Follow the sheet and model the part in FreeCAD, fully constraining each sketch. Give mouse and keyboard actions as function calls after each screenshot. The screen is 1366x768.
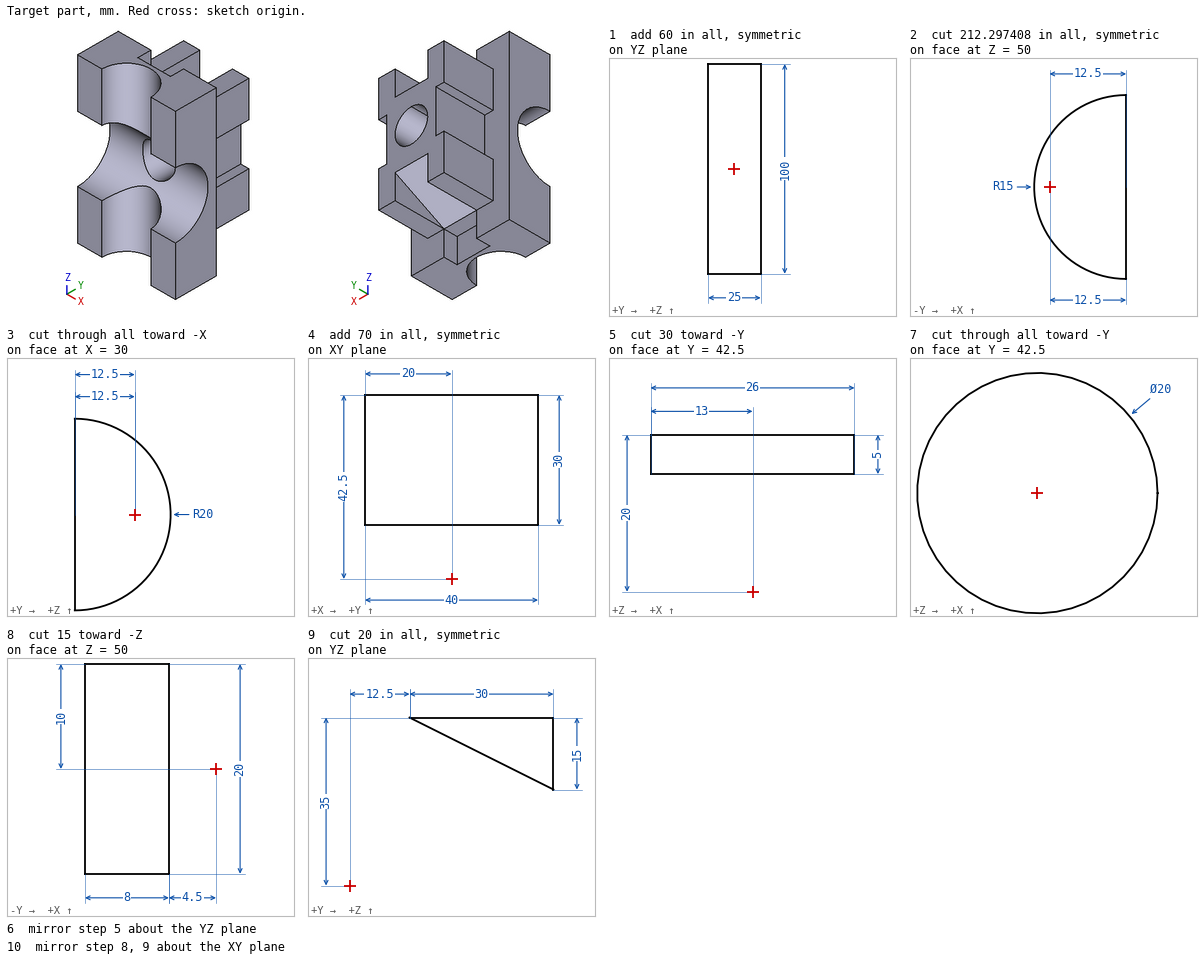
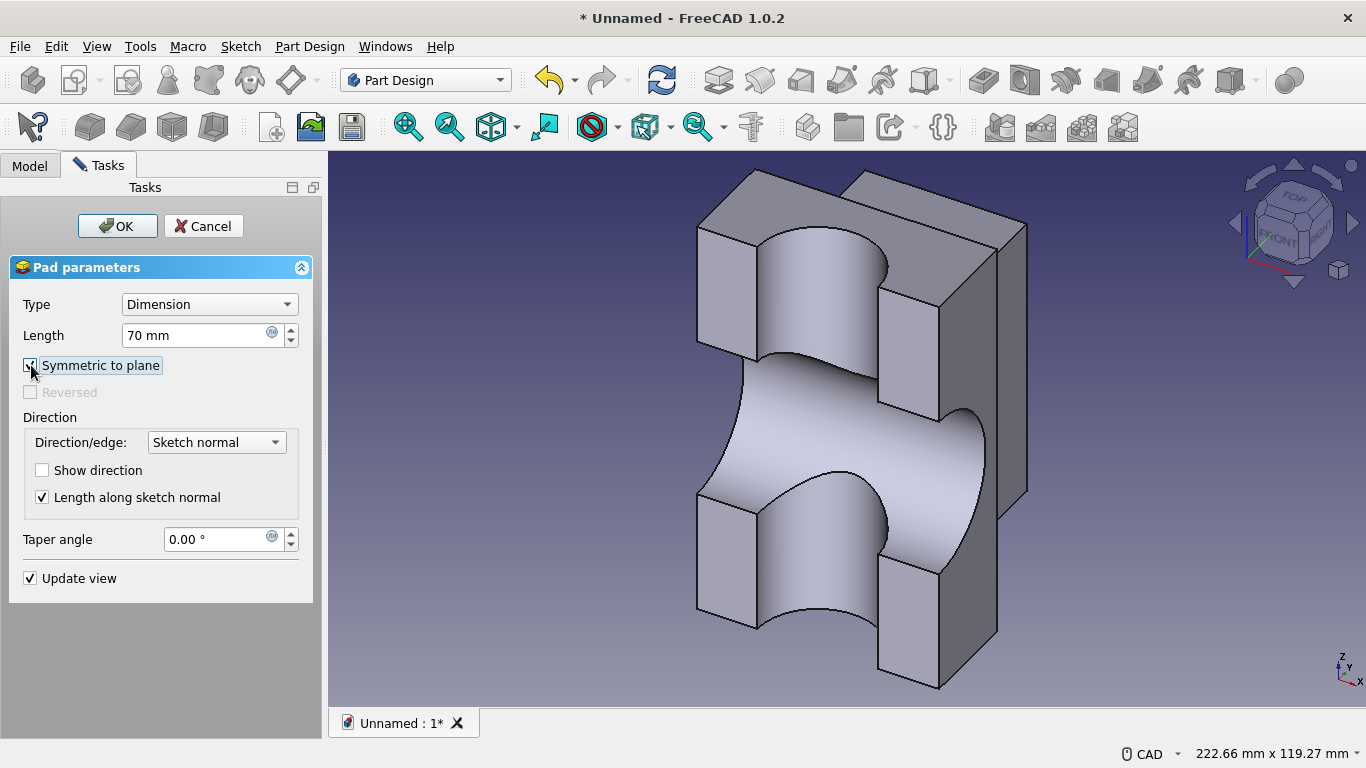
click(118, 226)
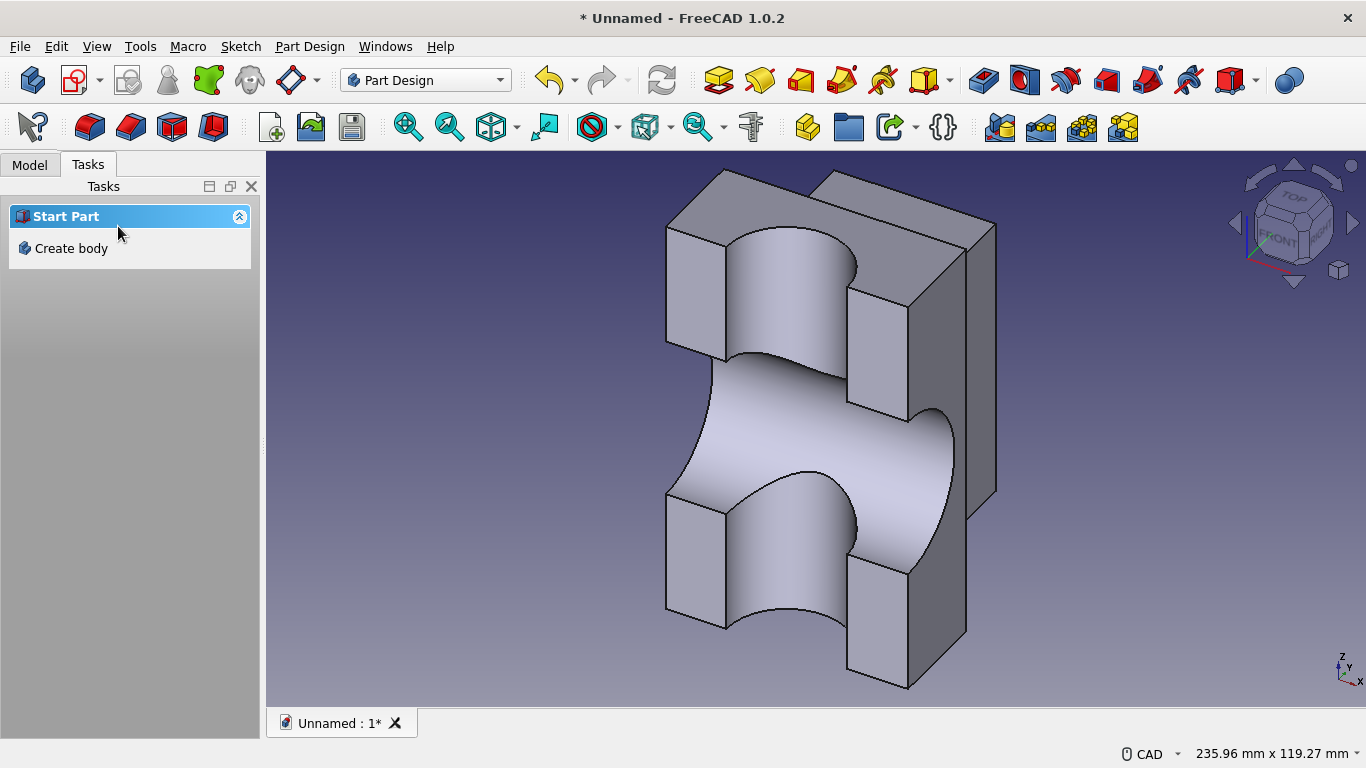
key(v)
key(f)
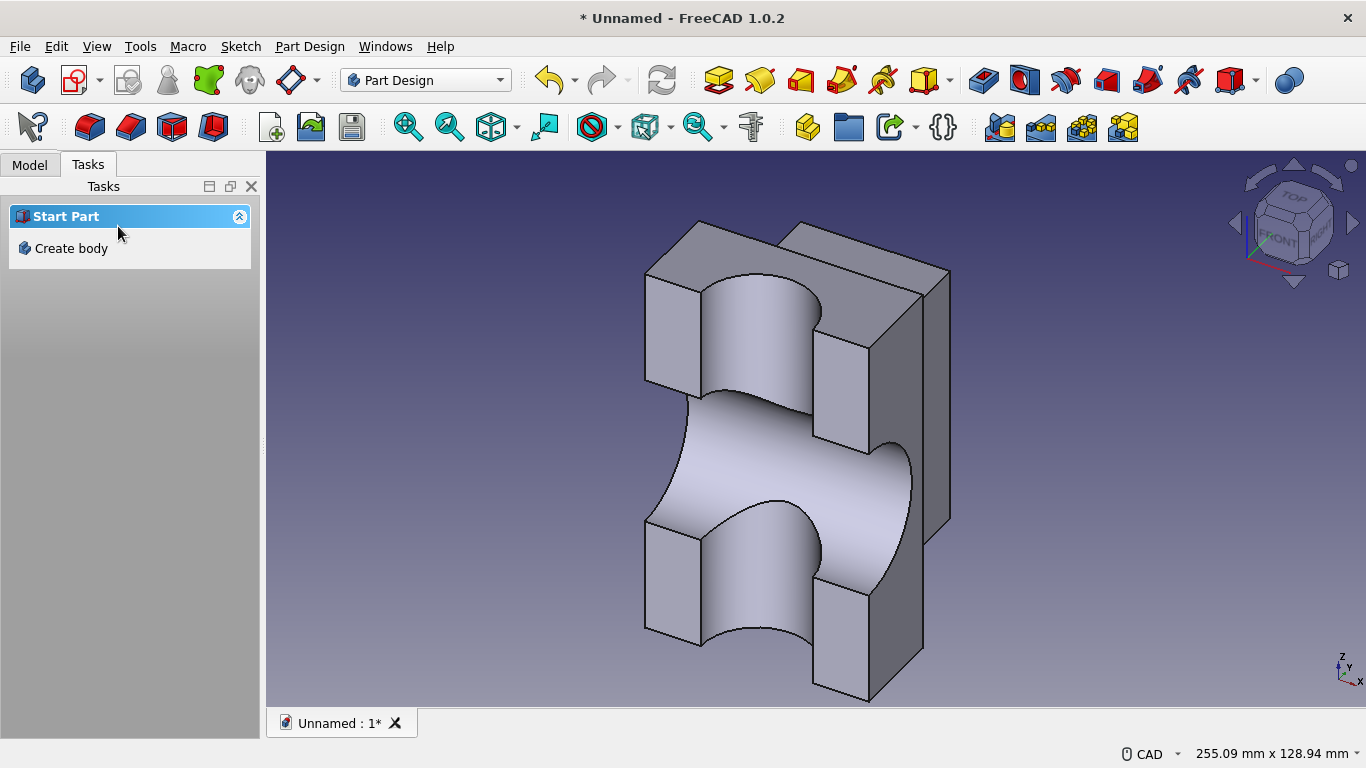
key(4)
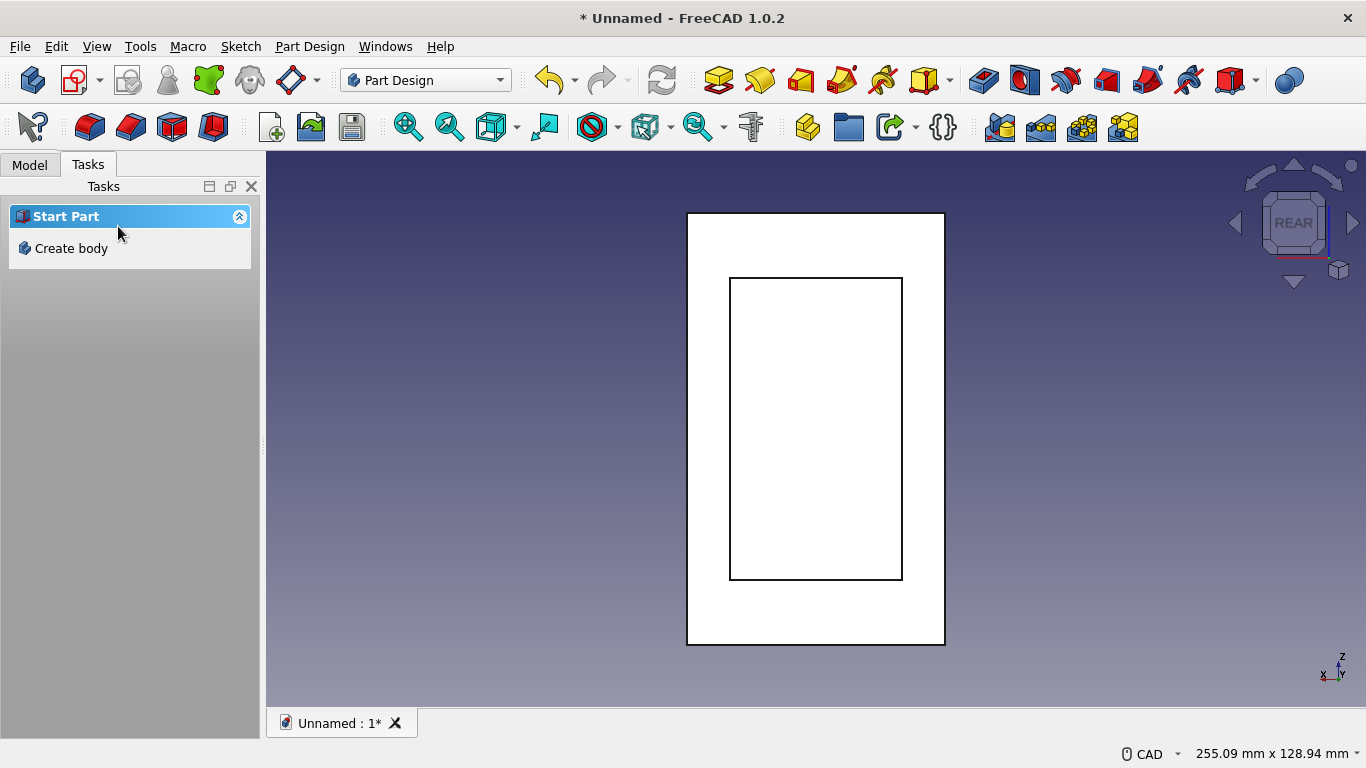
click(816, 428)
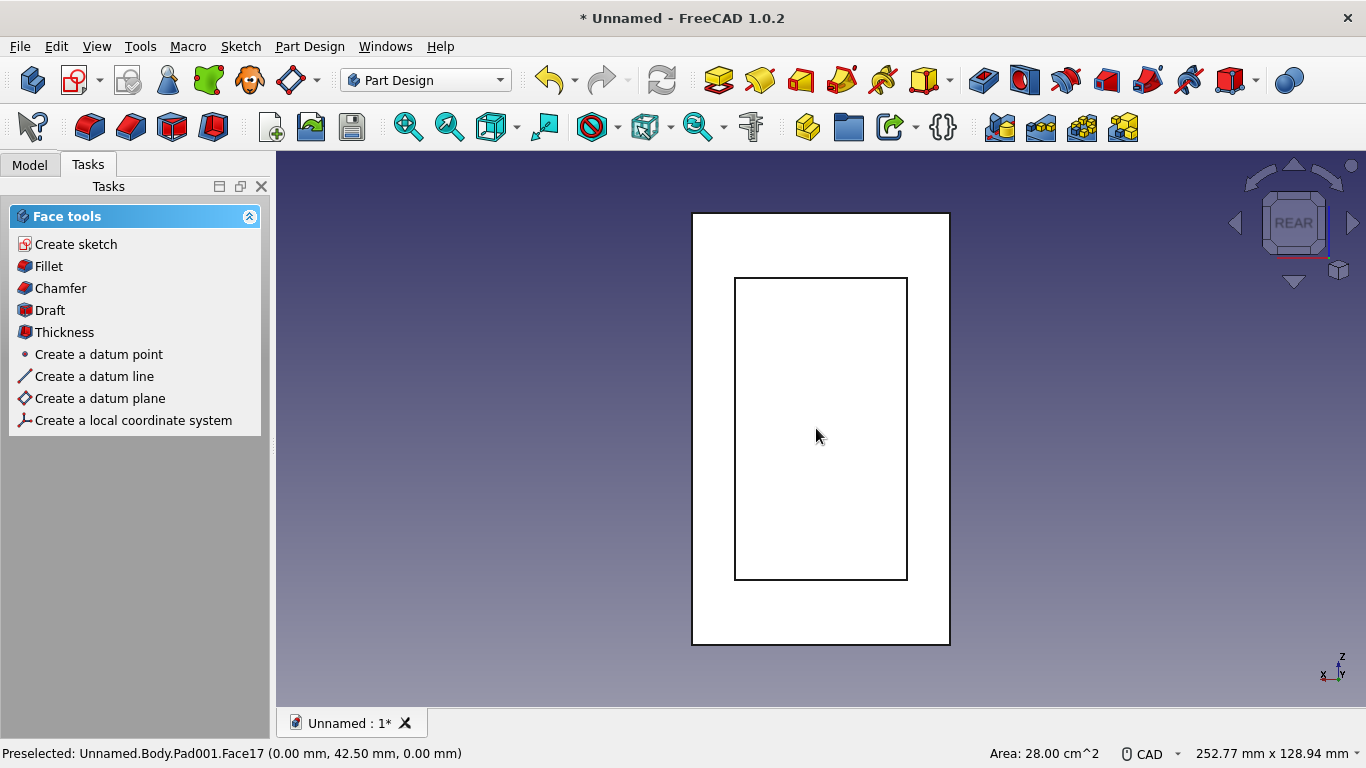
click(74, 80)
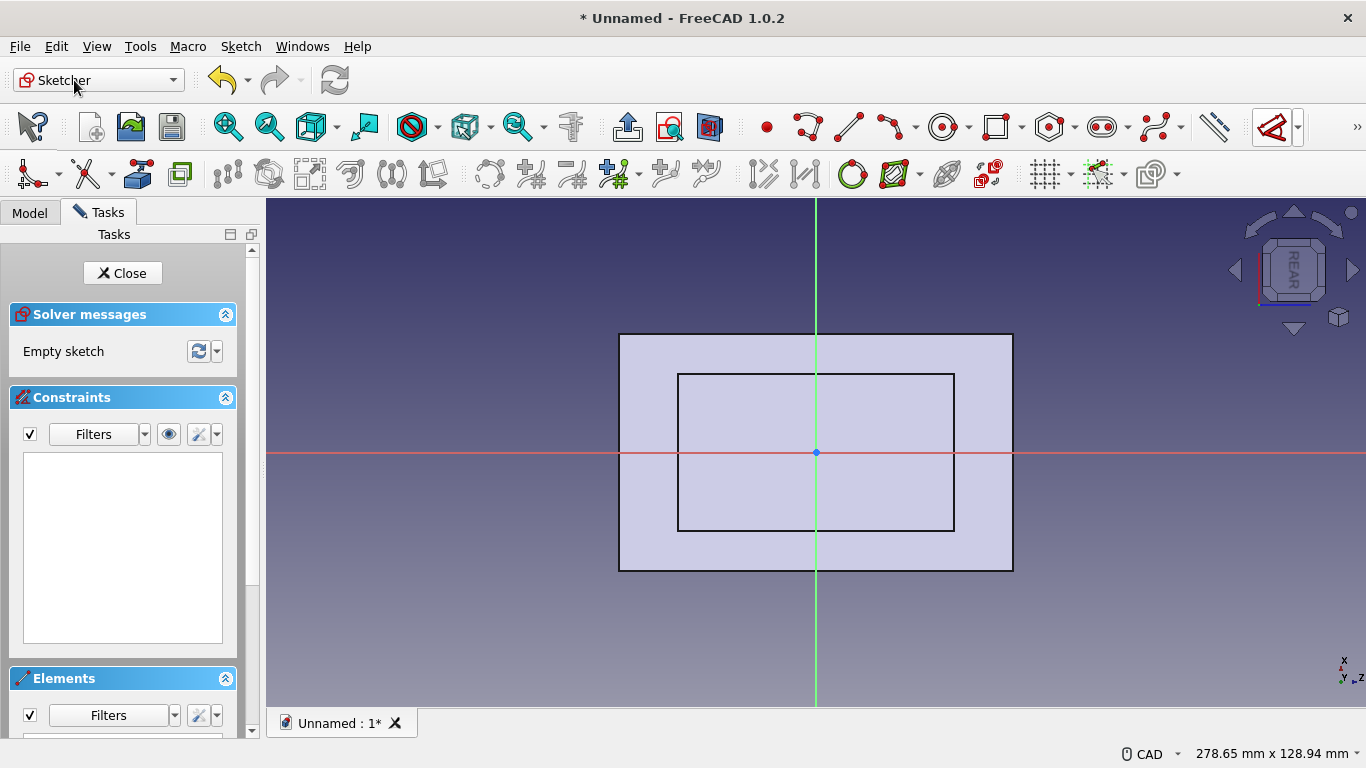
scroll(838, 400, up, 7)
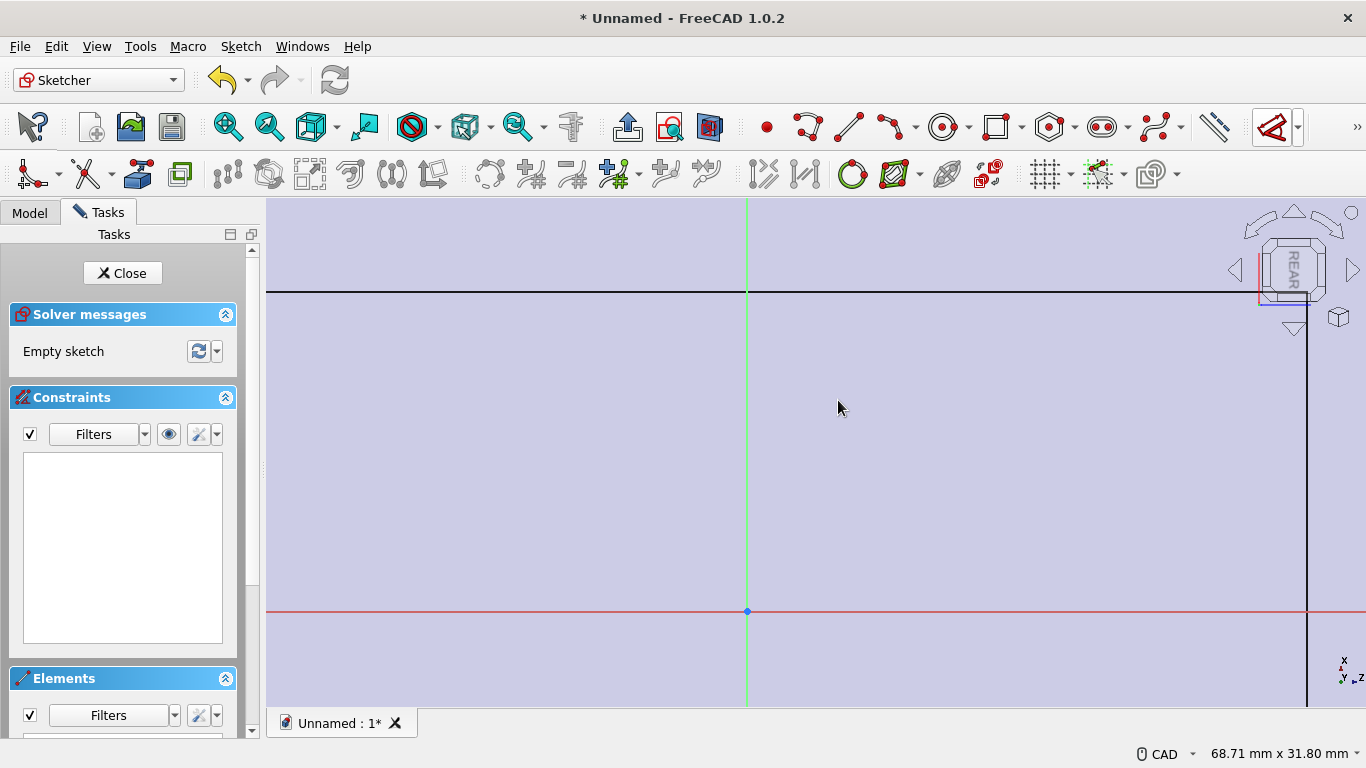
click(996, 128)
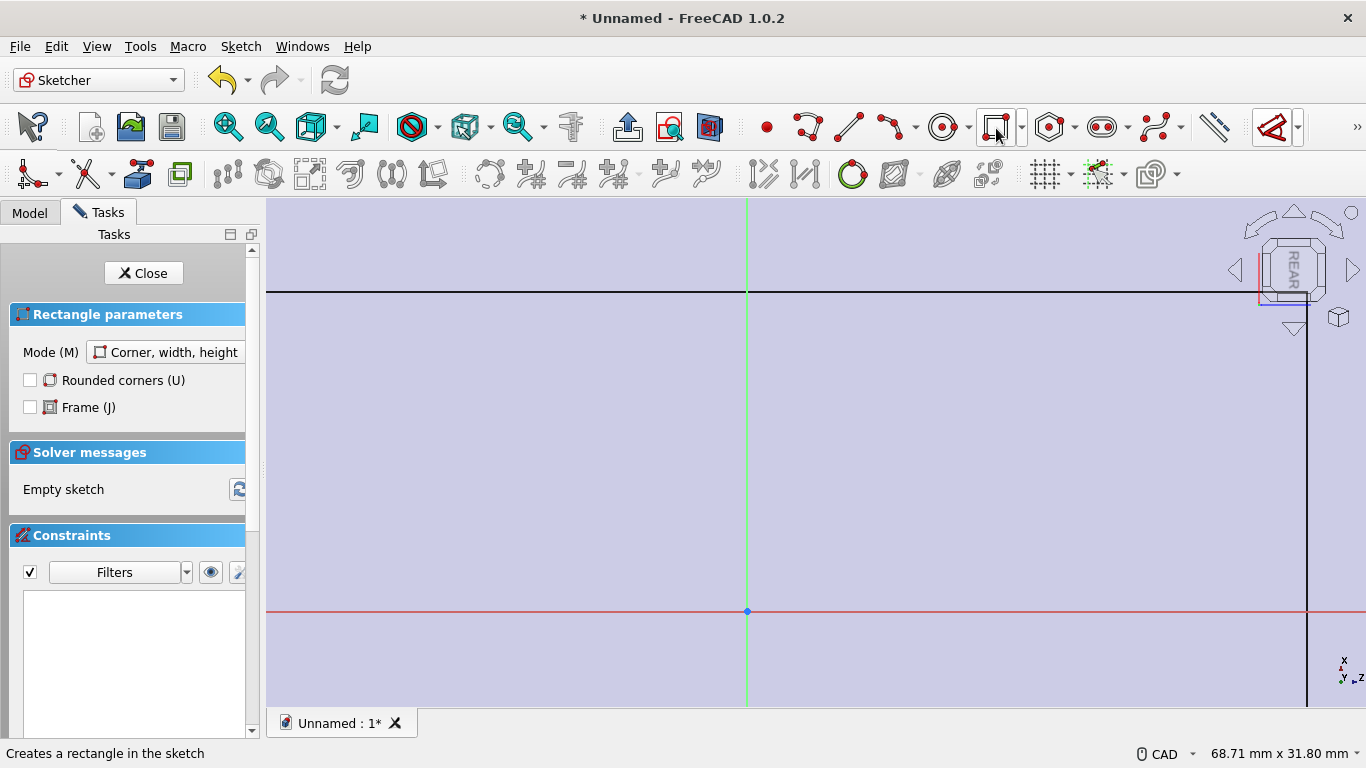
click(539, 292)
move(955, 372)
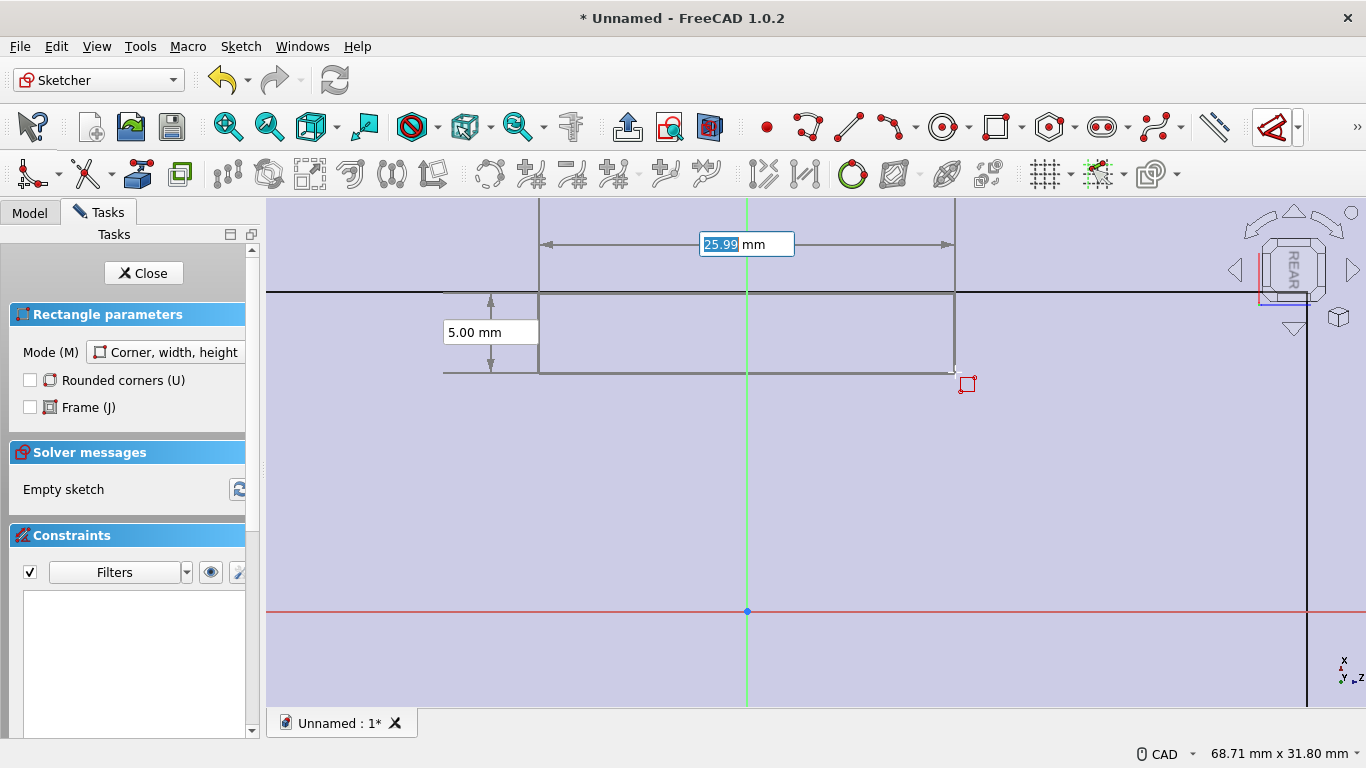
text(26)
key(Tab)
text(5)
key(Return)
key(Escape)